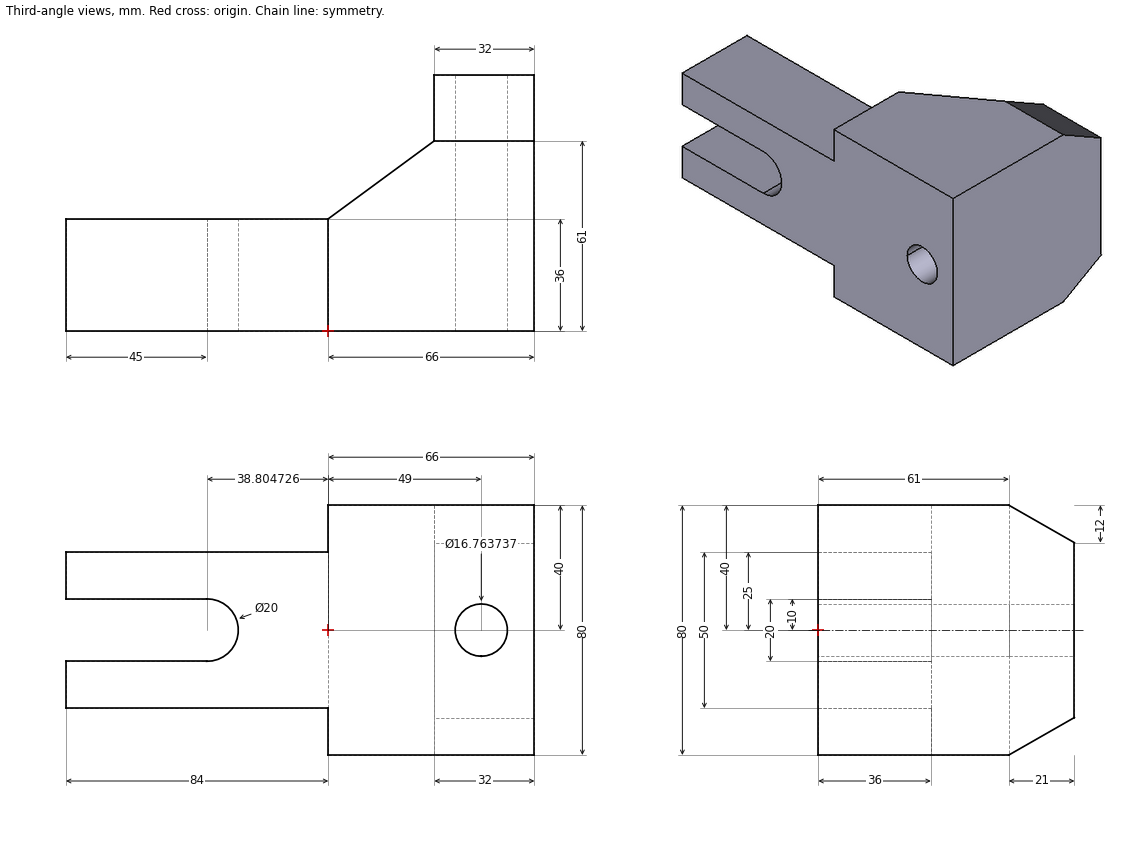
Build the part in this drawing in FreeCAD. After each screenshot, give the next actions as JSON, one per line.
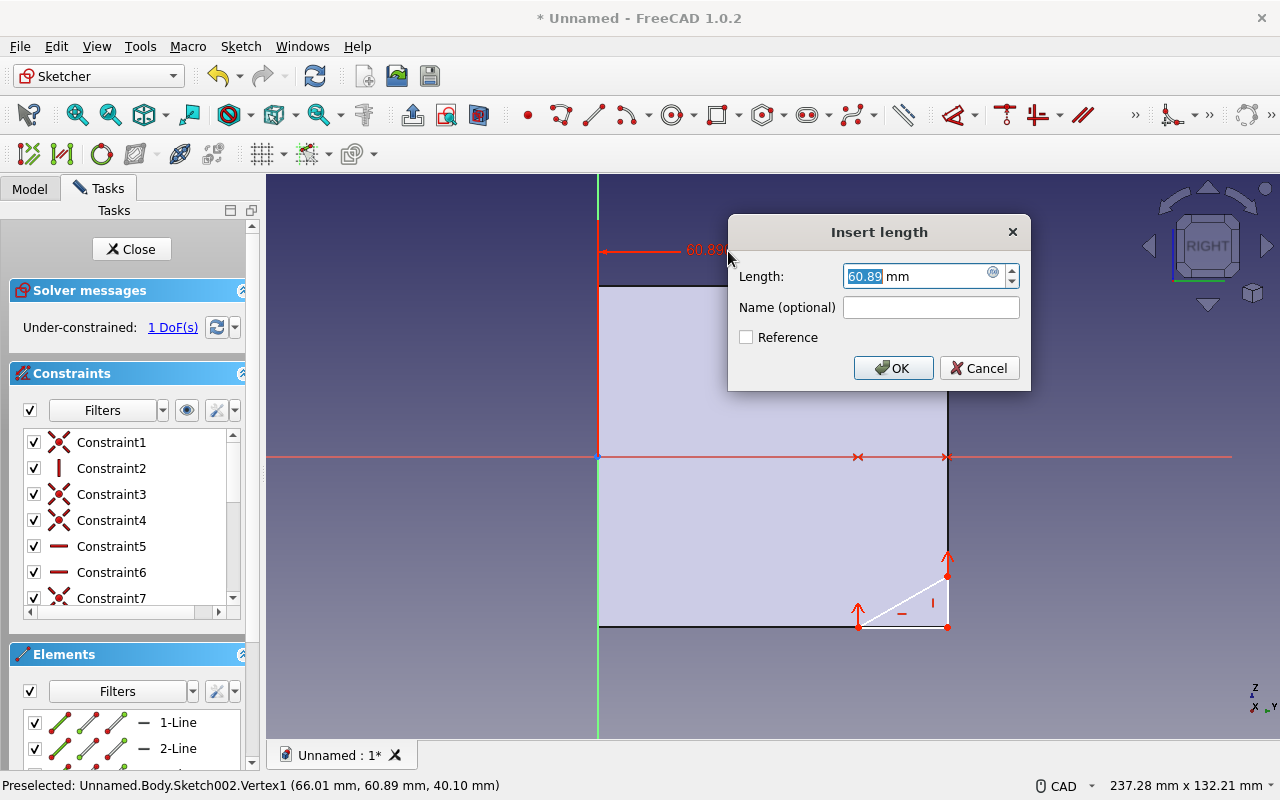
{"action": "type", "text": "61"}
{"action": "key", "text": "Return"}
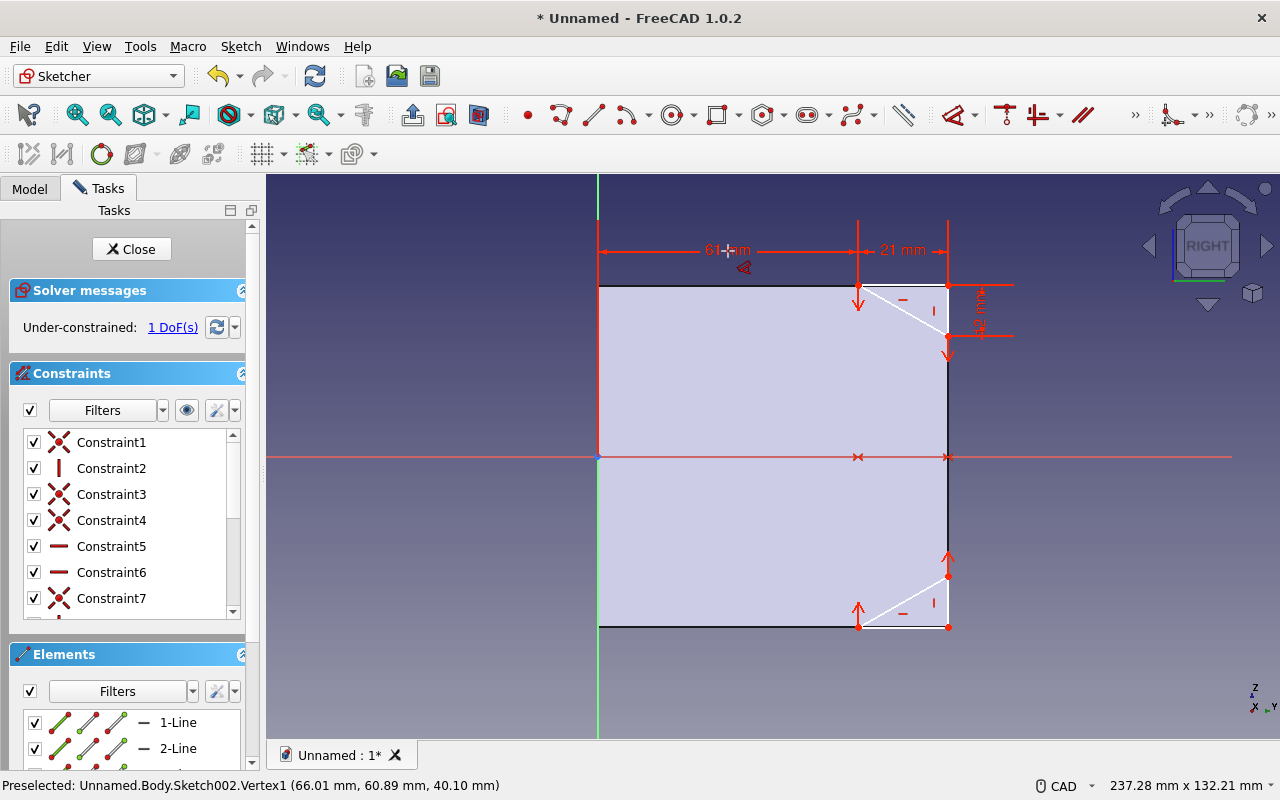
{"action": "left_click", "coordinate": [858, 285]}
{"action": "left_click", "coordinate": [564, 371]}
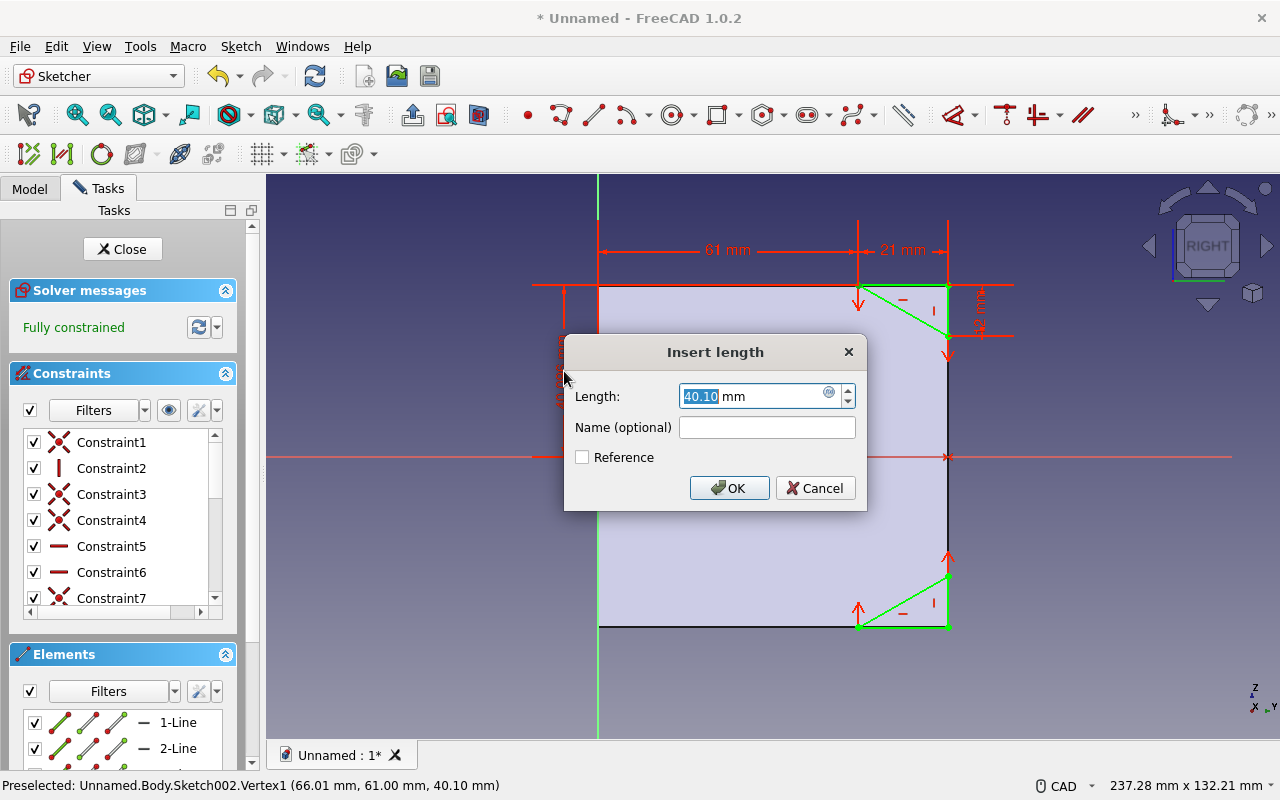
{"action": "type", "text": "40"}
{"action": "key", "text": "Return"}
{"action": "key", "text": "Escape"}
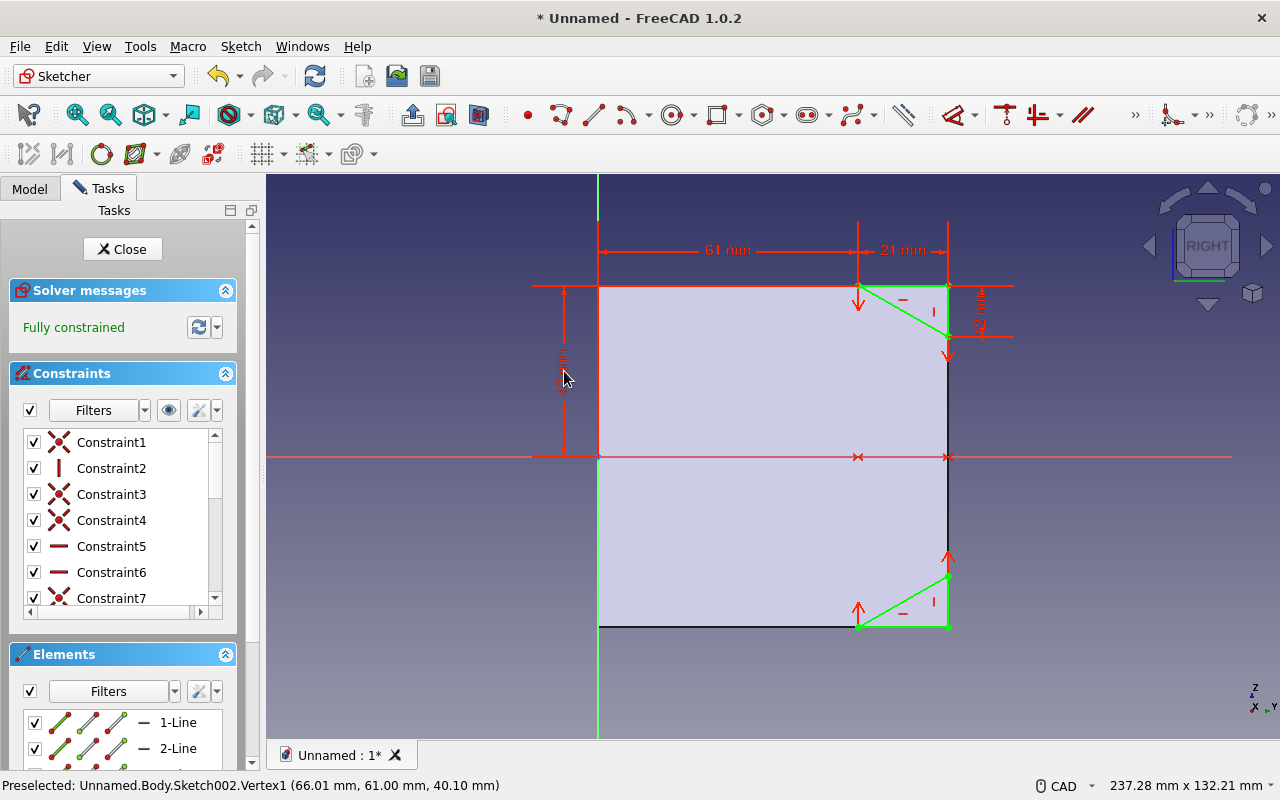
{"action": "left_click", "coordinate": [123, 249]}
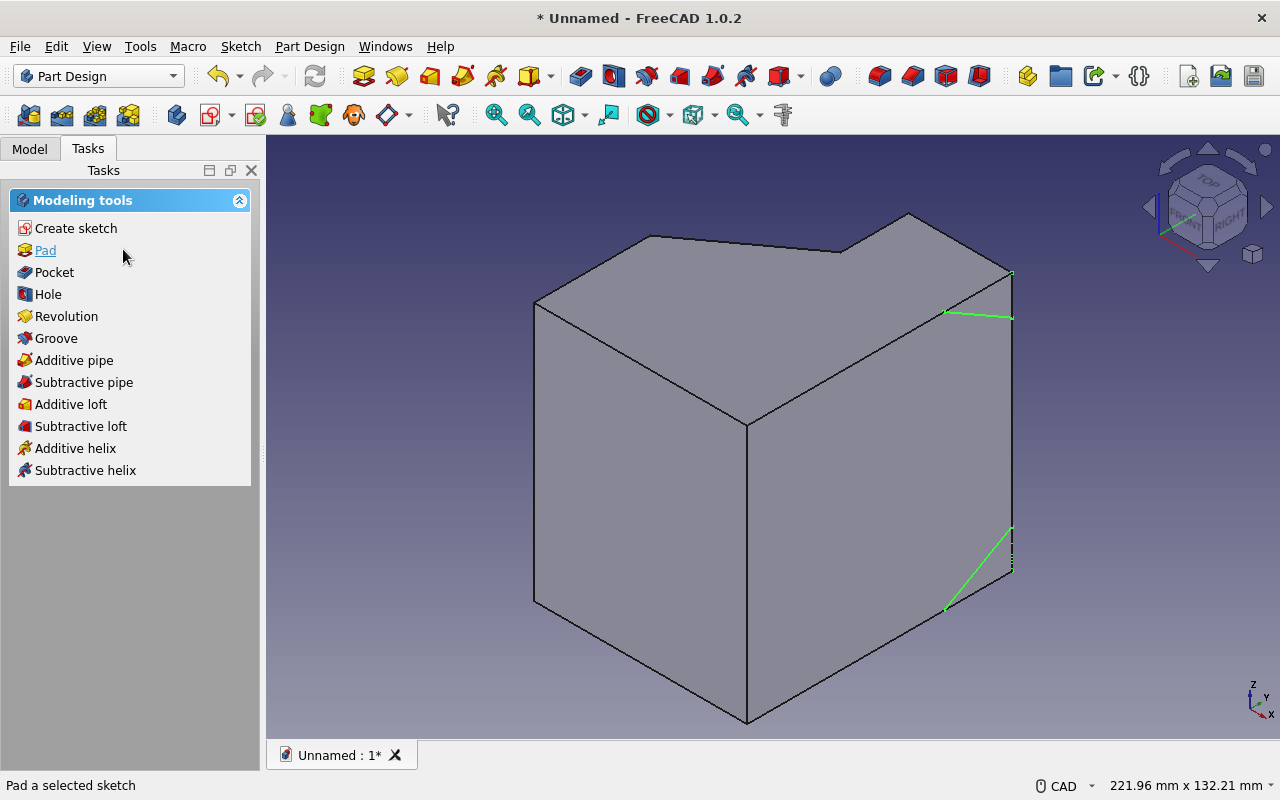
{"action": "left_click", "coordinate": [581, 76]}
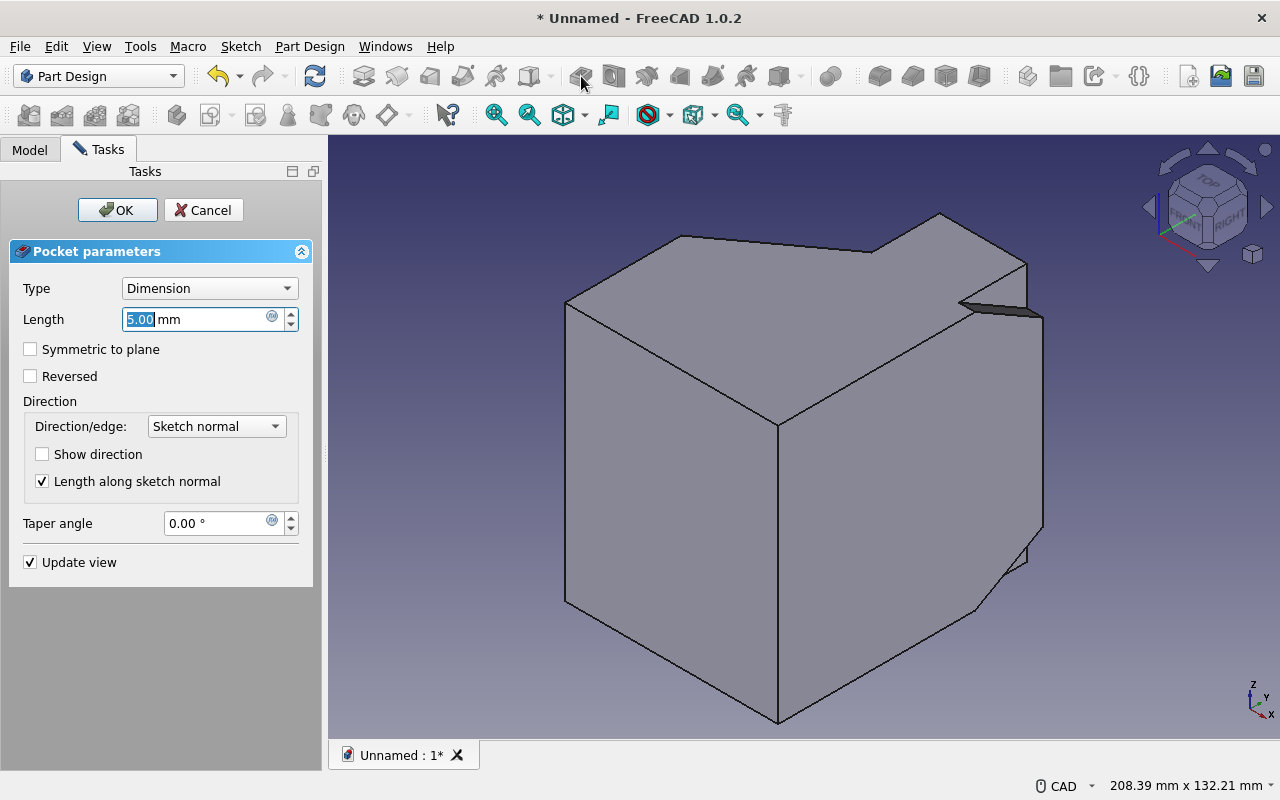
{"action": "type", "text": "32"}
{"action": "key", "text": "Tab"}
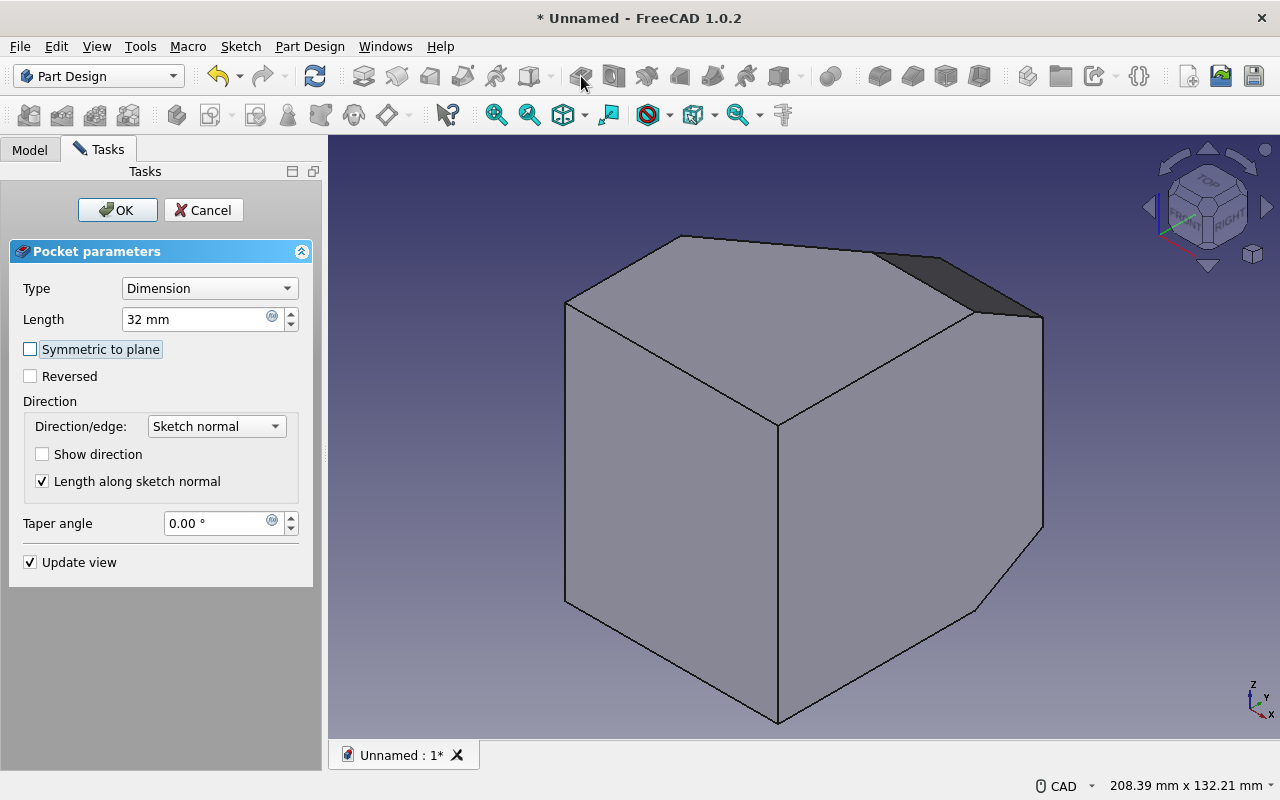
{"action": "left_click", "coordinate": [118, 210]}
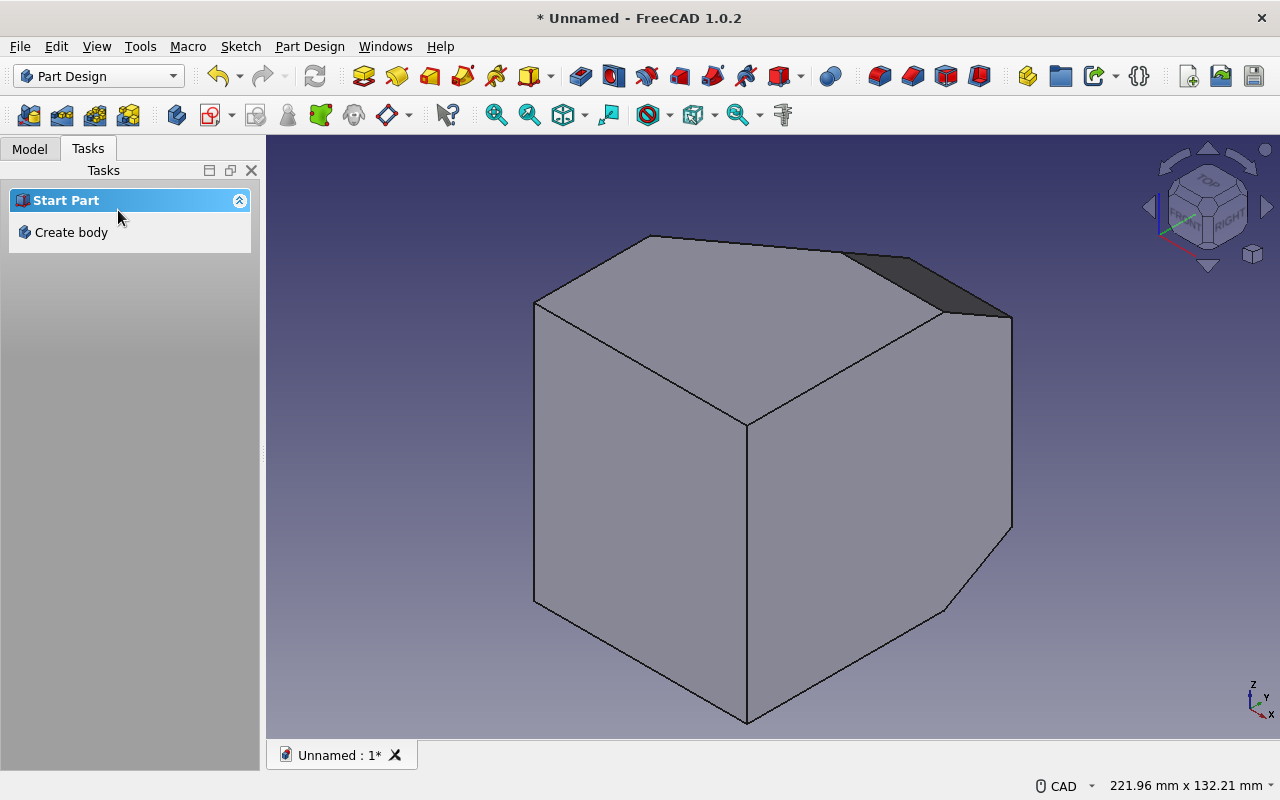
{"action": "left_click", "coordinate": [210, 116]}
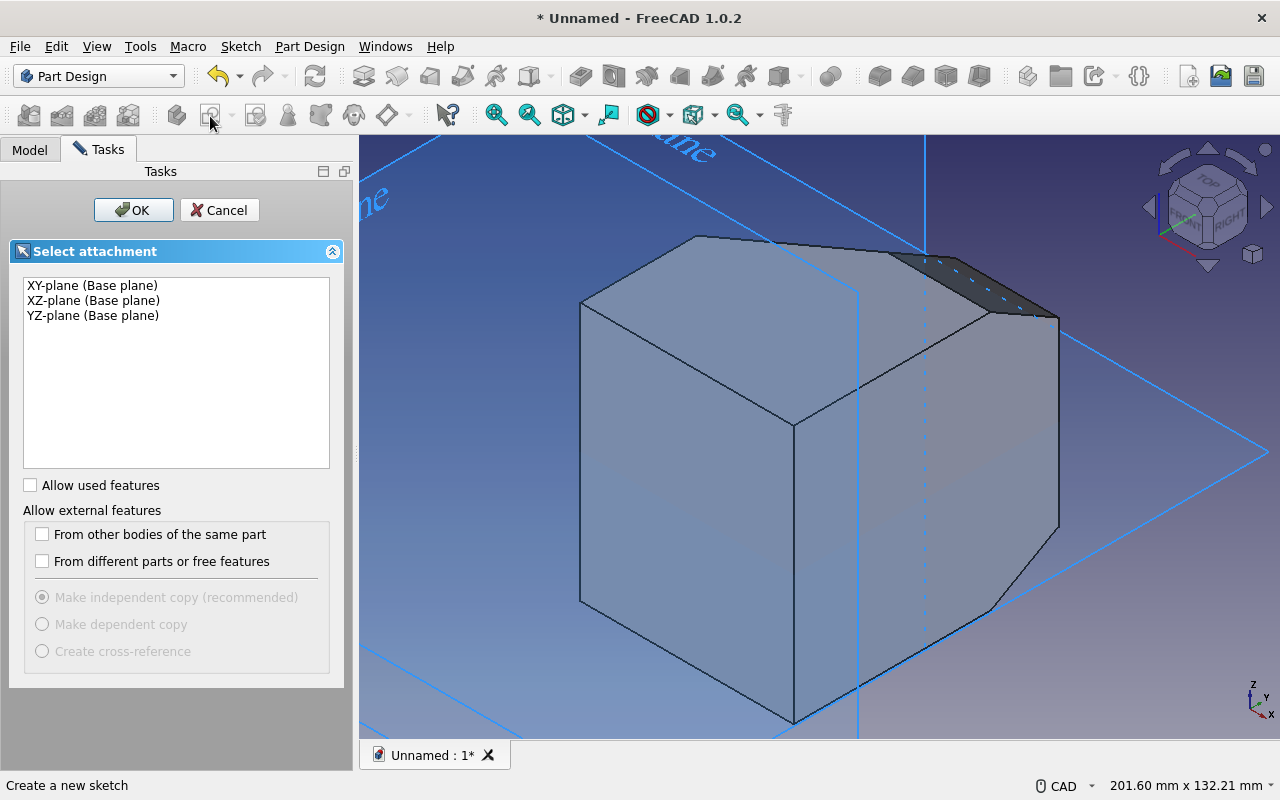
{"action": "left_click", "coordinate": [84, 316]}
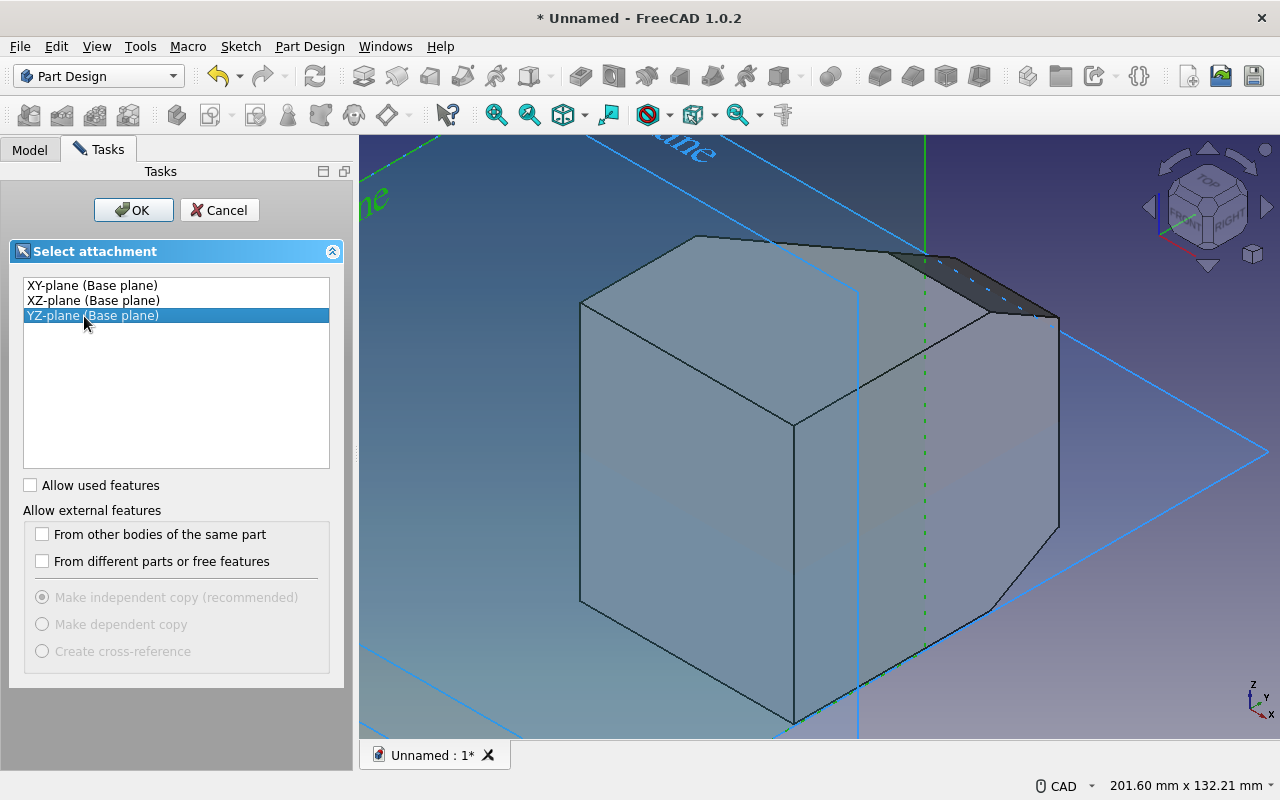
{"action": "left_click", "coordinate": [134, 210]}